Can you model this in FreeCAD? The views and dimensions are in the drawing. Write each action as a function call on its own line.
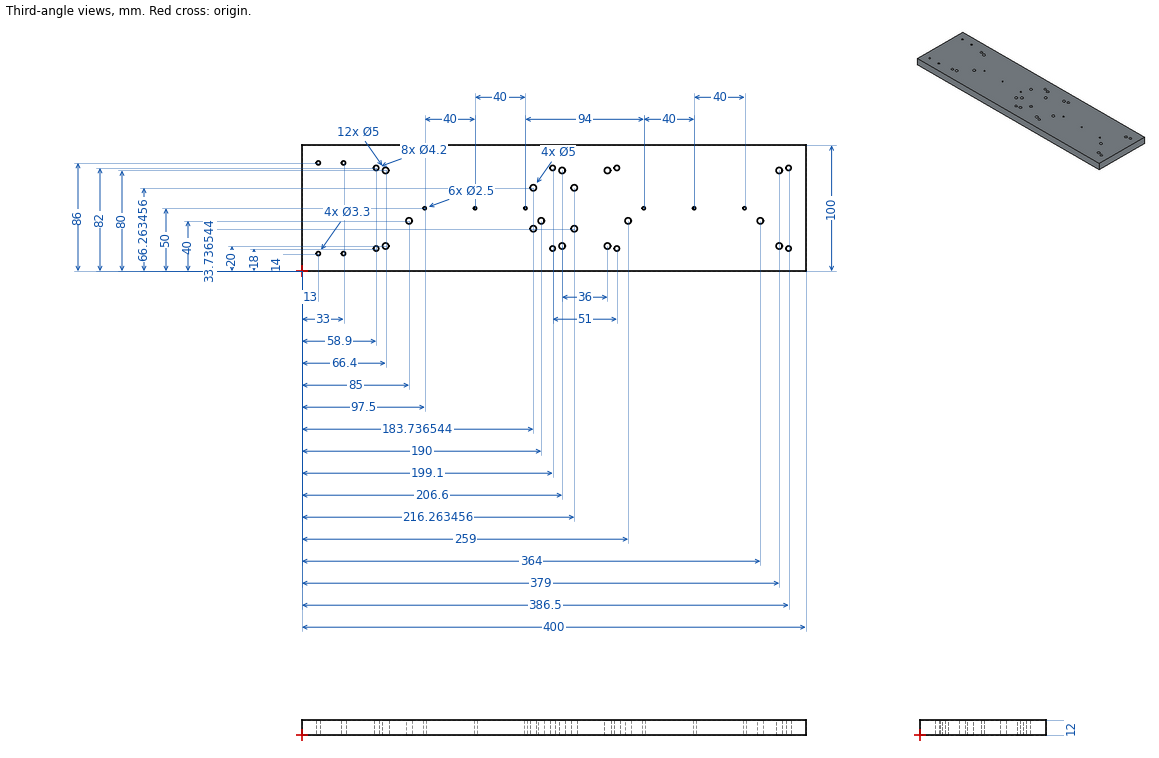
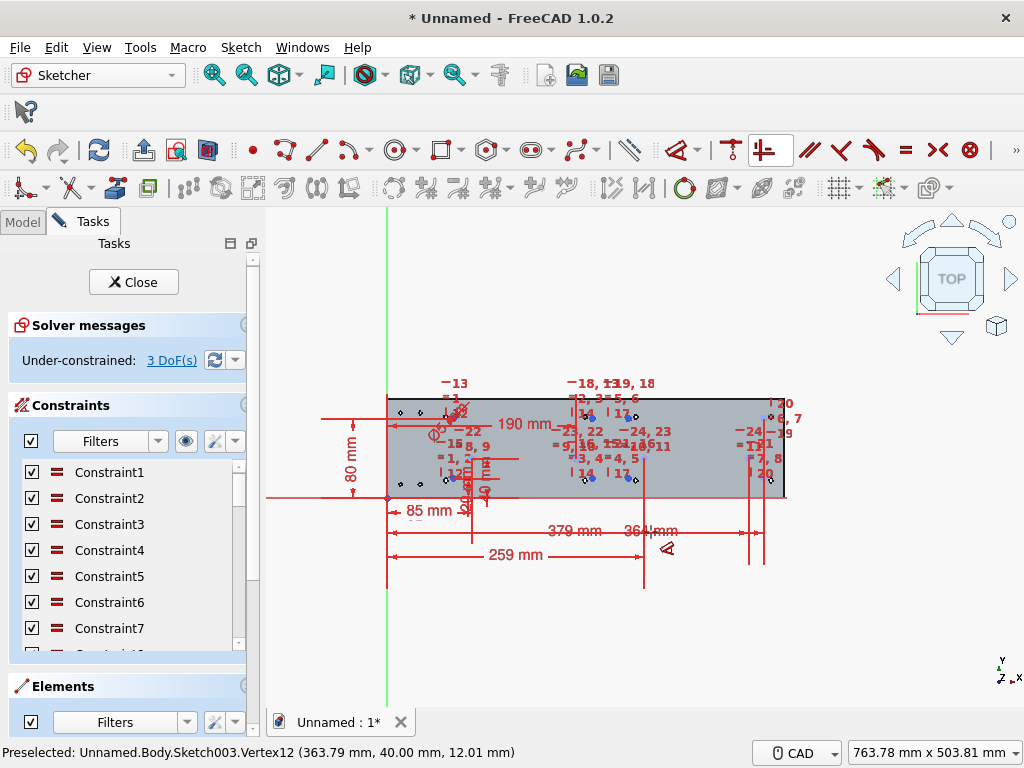
click(592, 479)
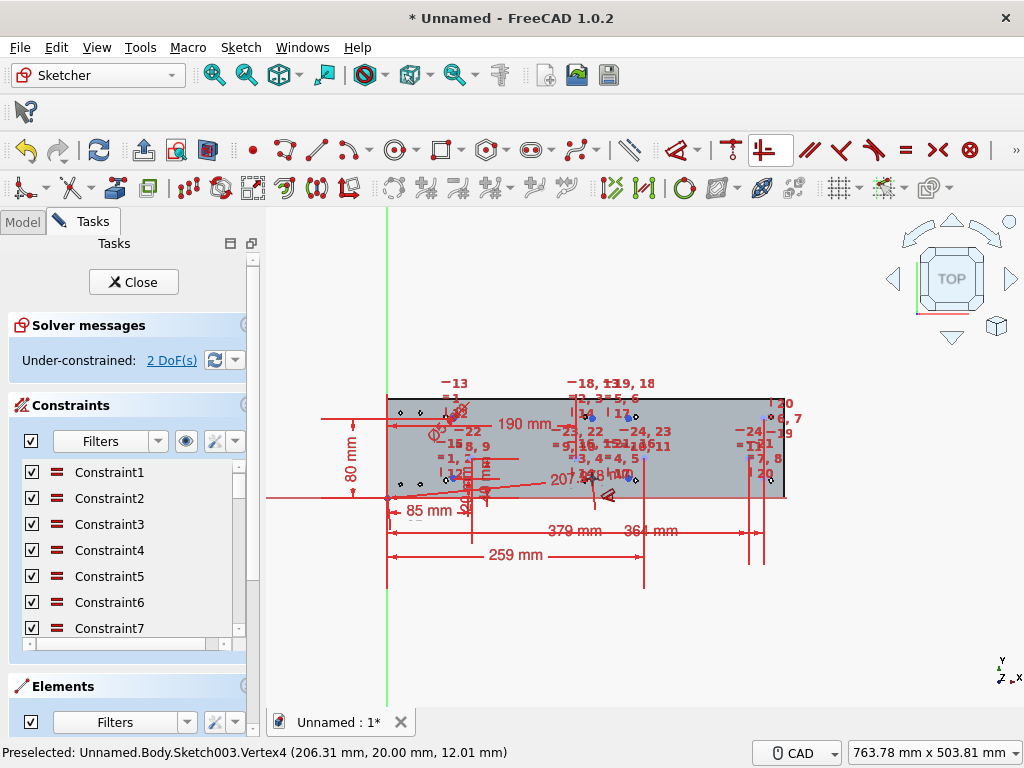
click(628, 479)
click(610, 445)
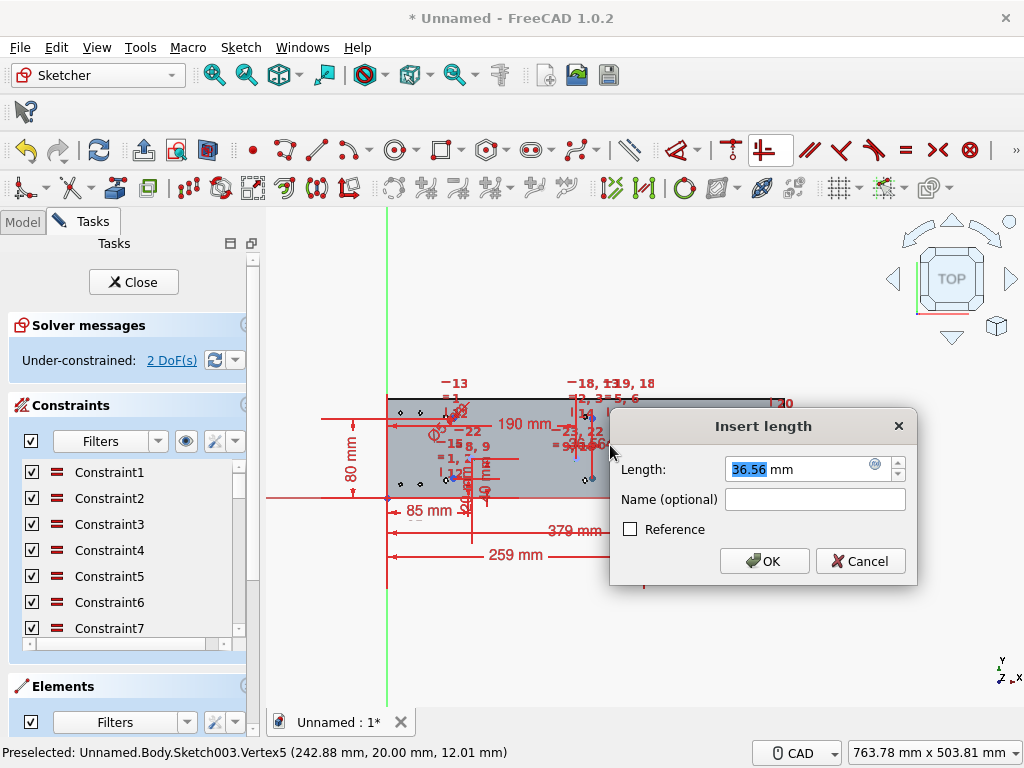
text(36)
key(Return)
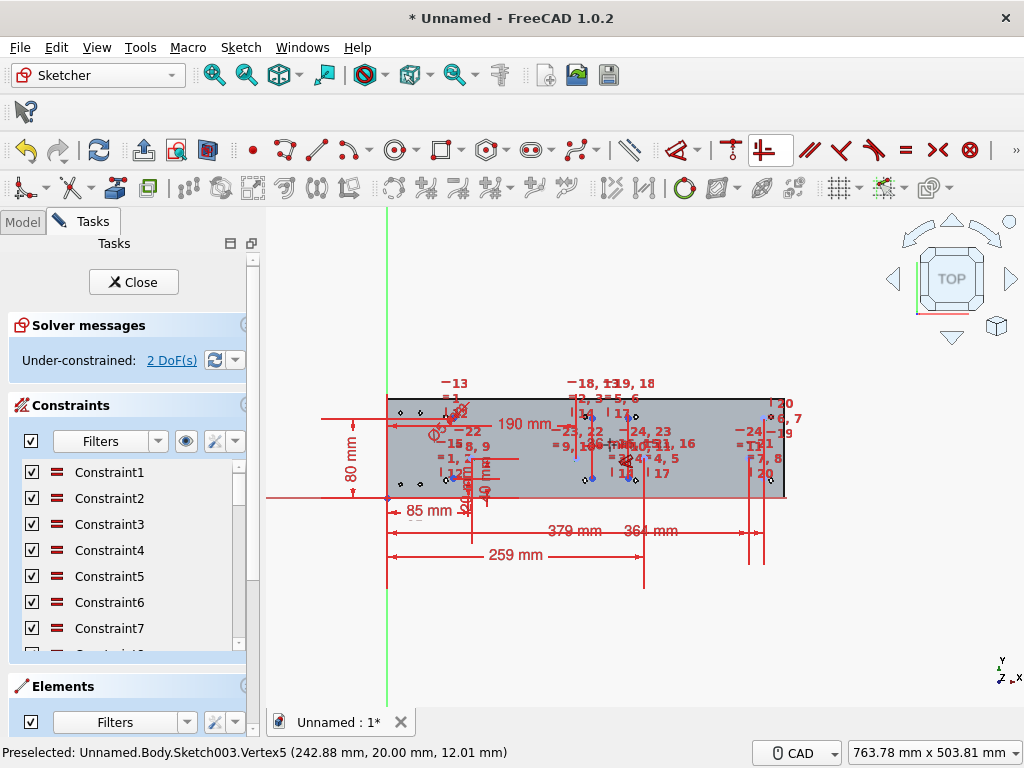
click(453, 419)
click(420, 385)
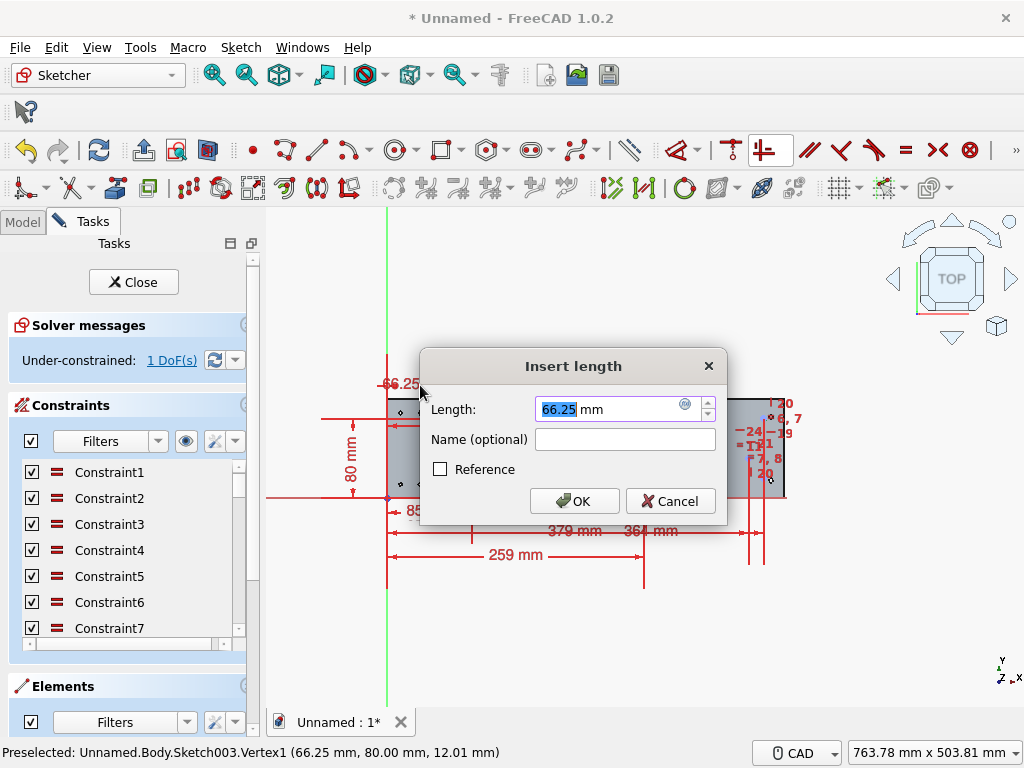
text(66.4)
key(Return)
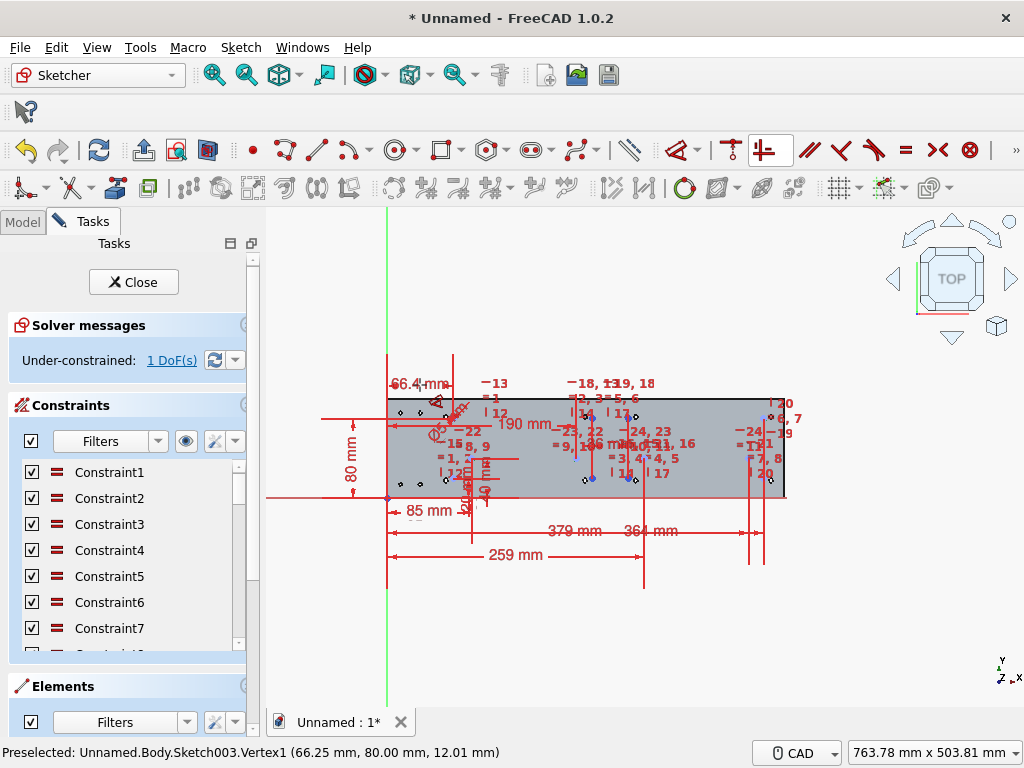
click(592, 419)
click(537, 385)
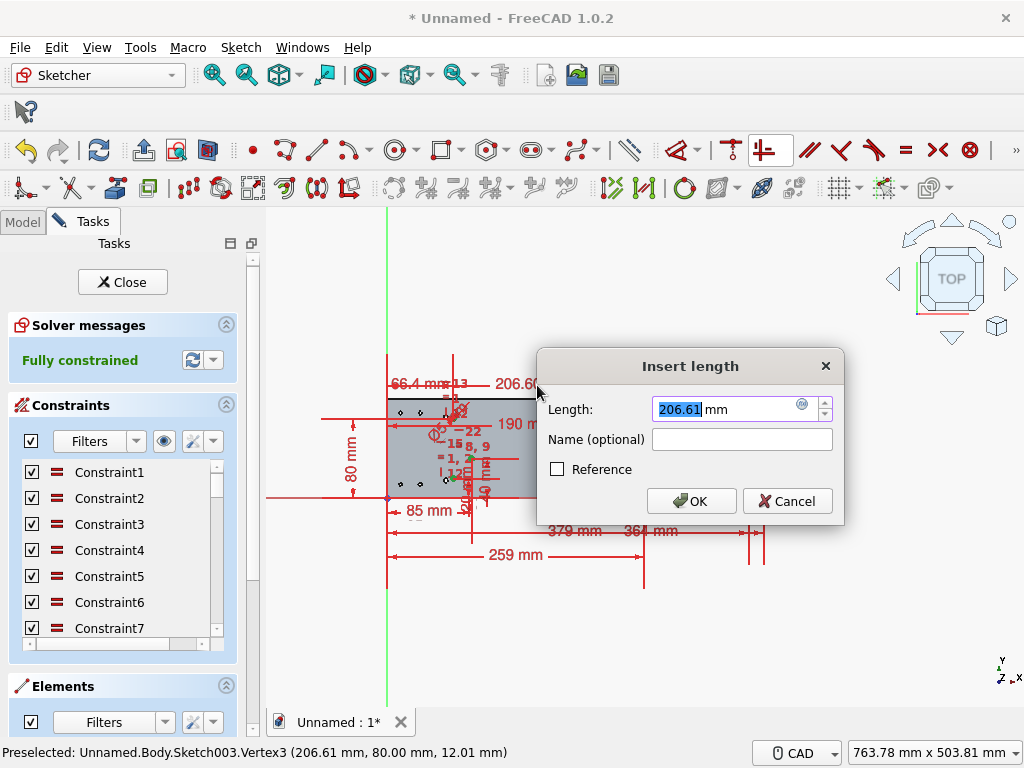
text(206.6)
key(Return)
key(Escape)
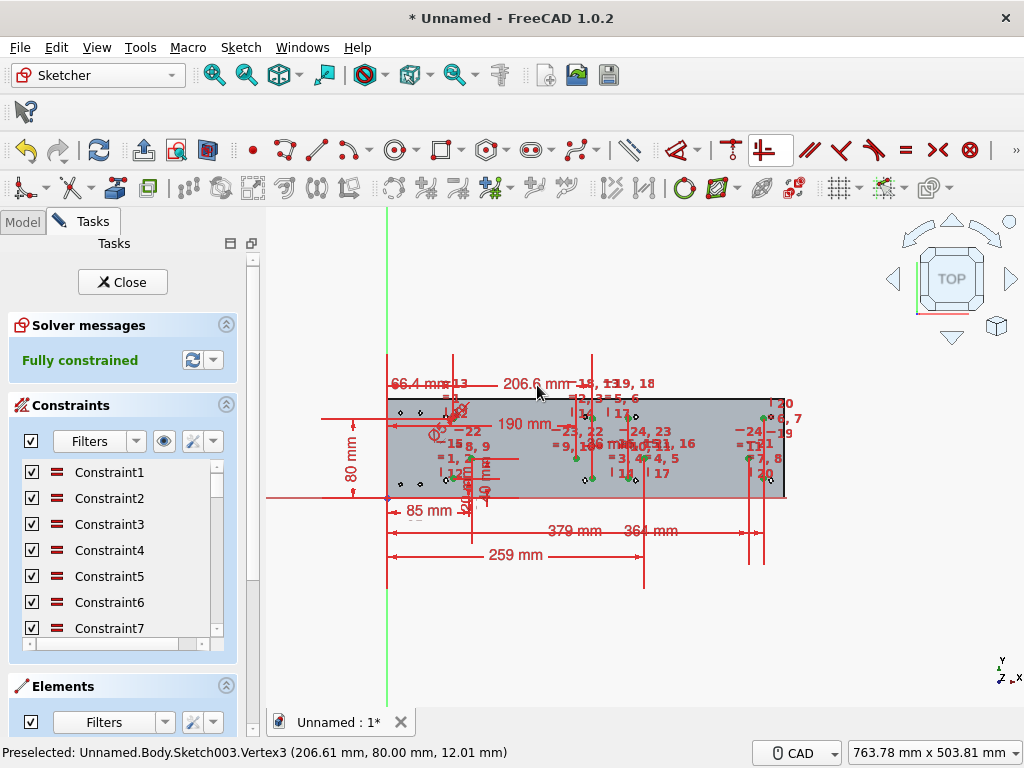
click(123, 282)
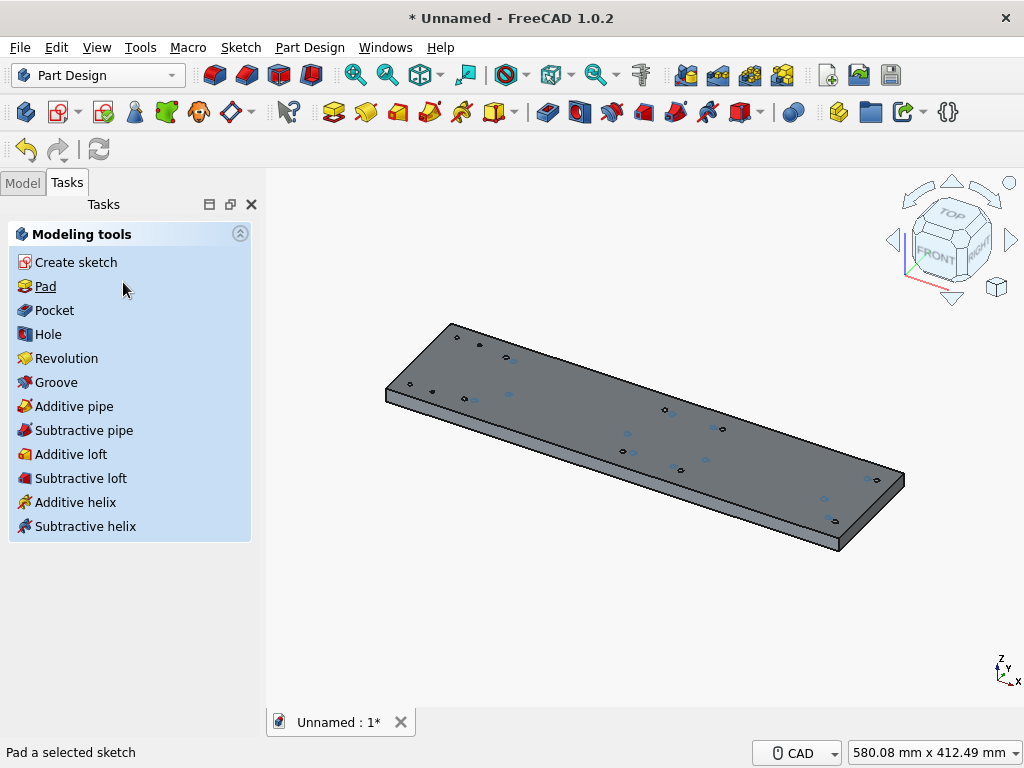
click(548, 112)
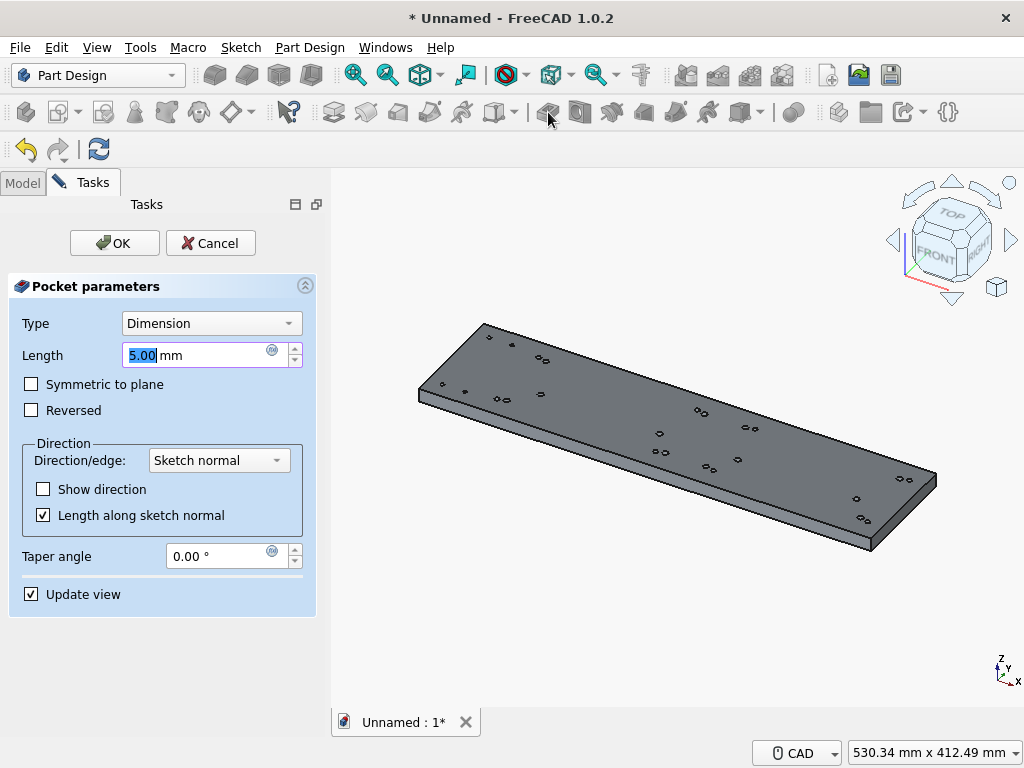
click(212, 324)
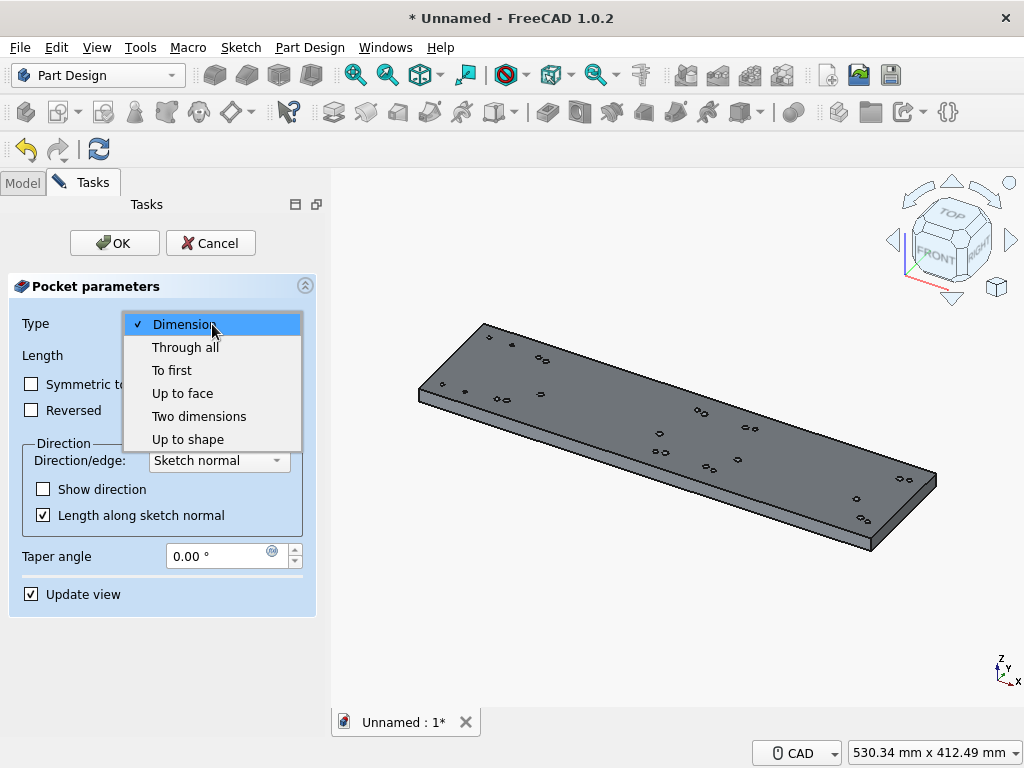
click(212, 348)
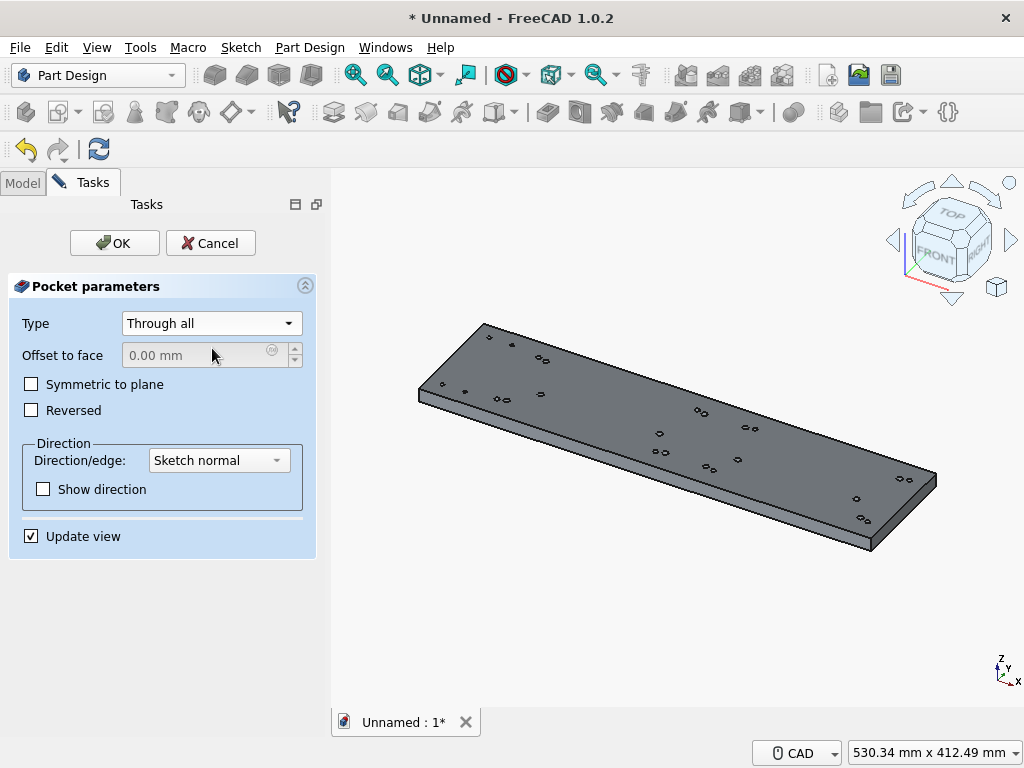
click(115, 243)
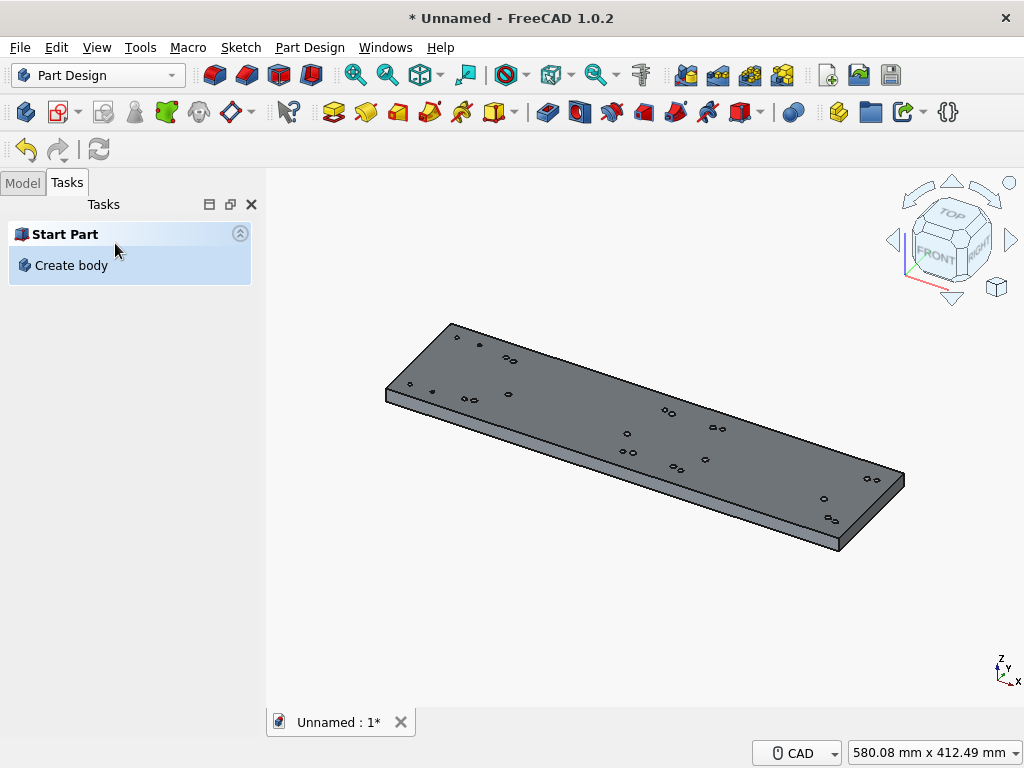
click(774, 473)